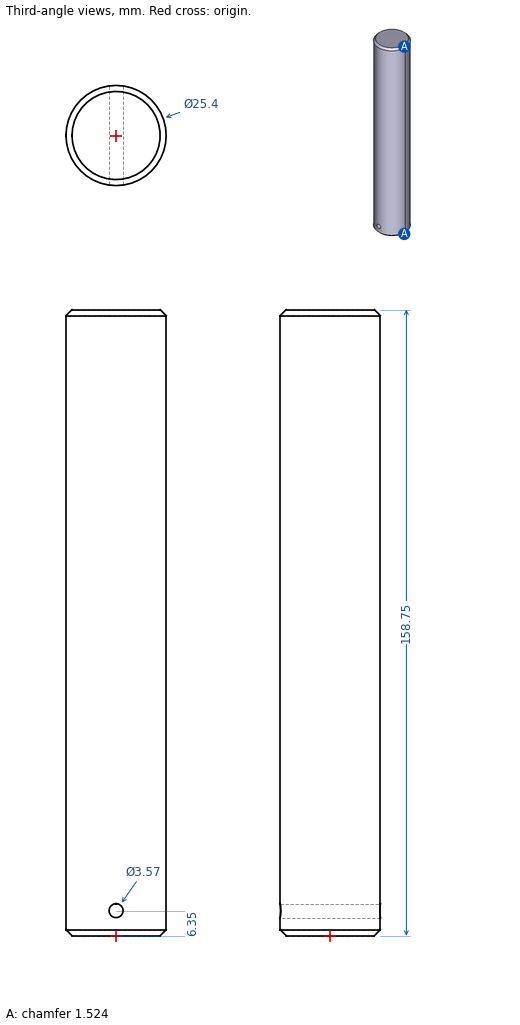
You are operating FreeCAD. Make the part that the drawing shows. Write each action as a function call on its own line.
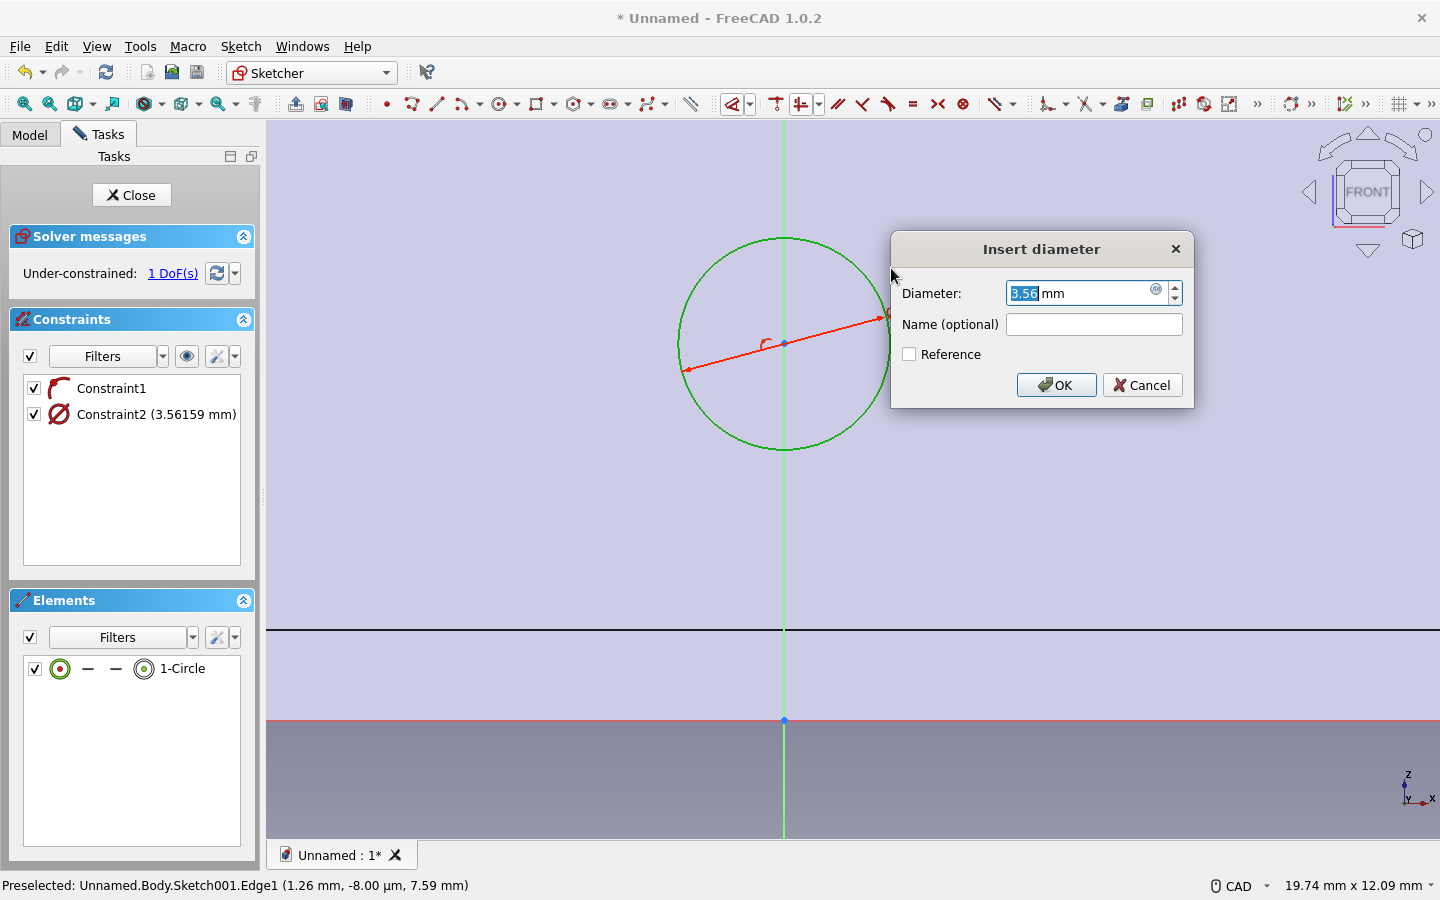
text(3.57)
key(Return)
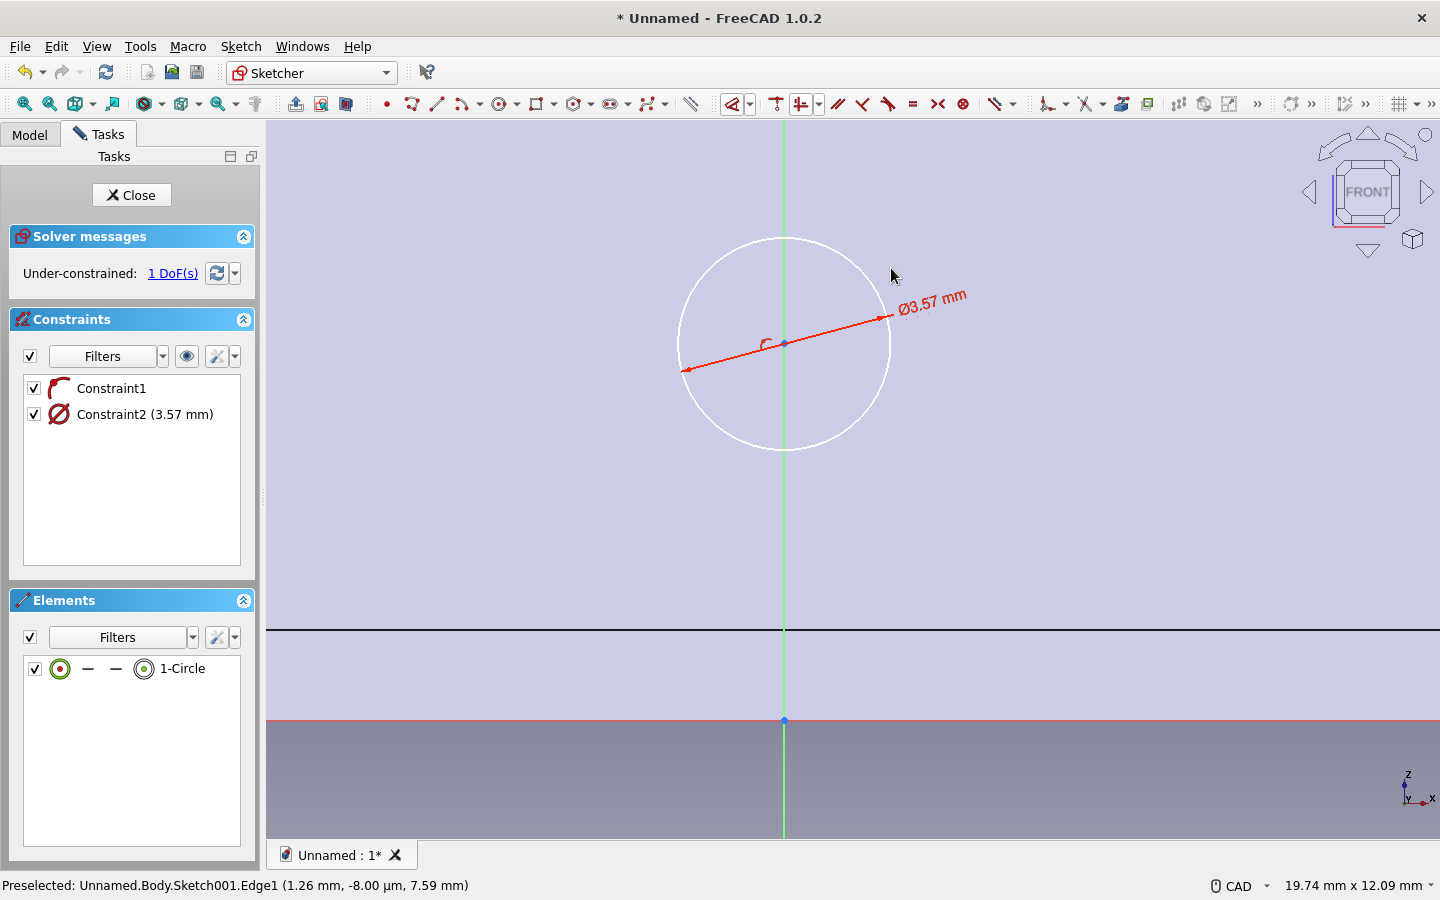
click(784, 344)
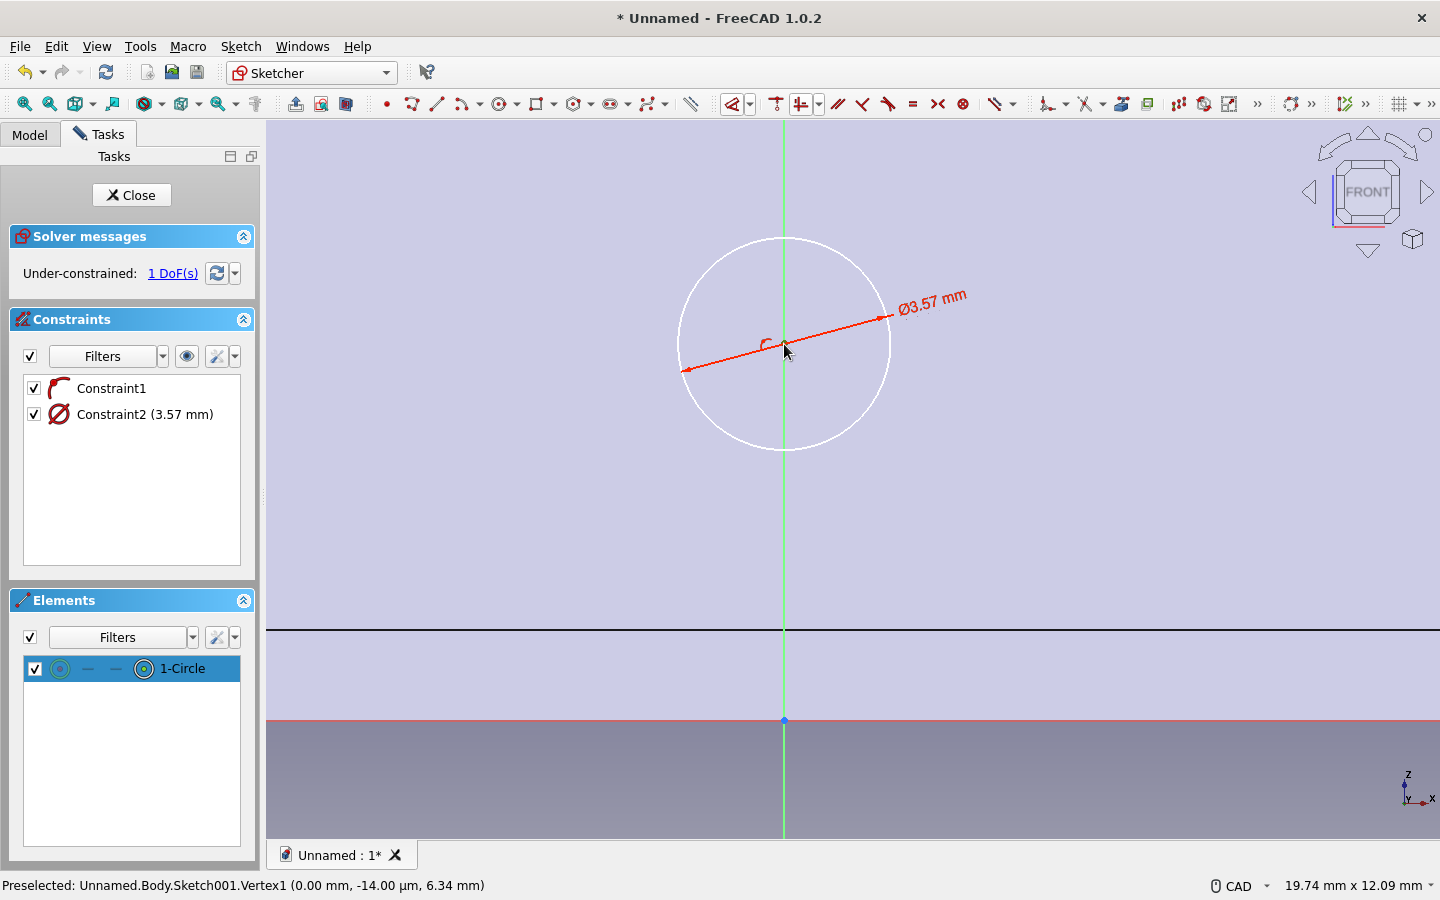
key(i)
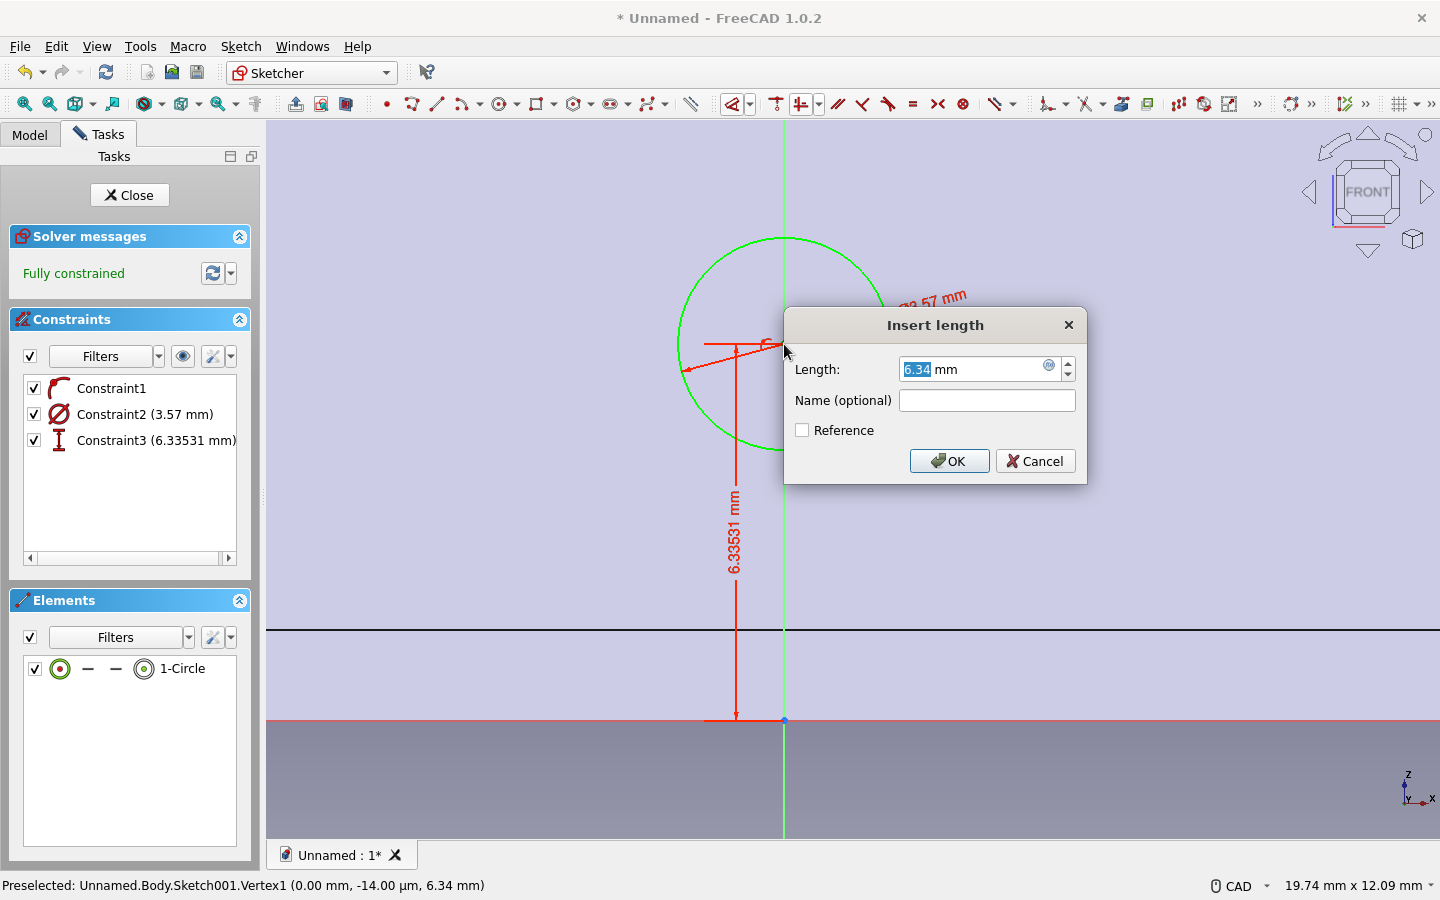
text(6.35)
key(Return)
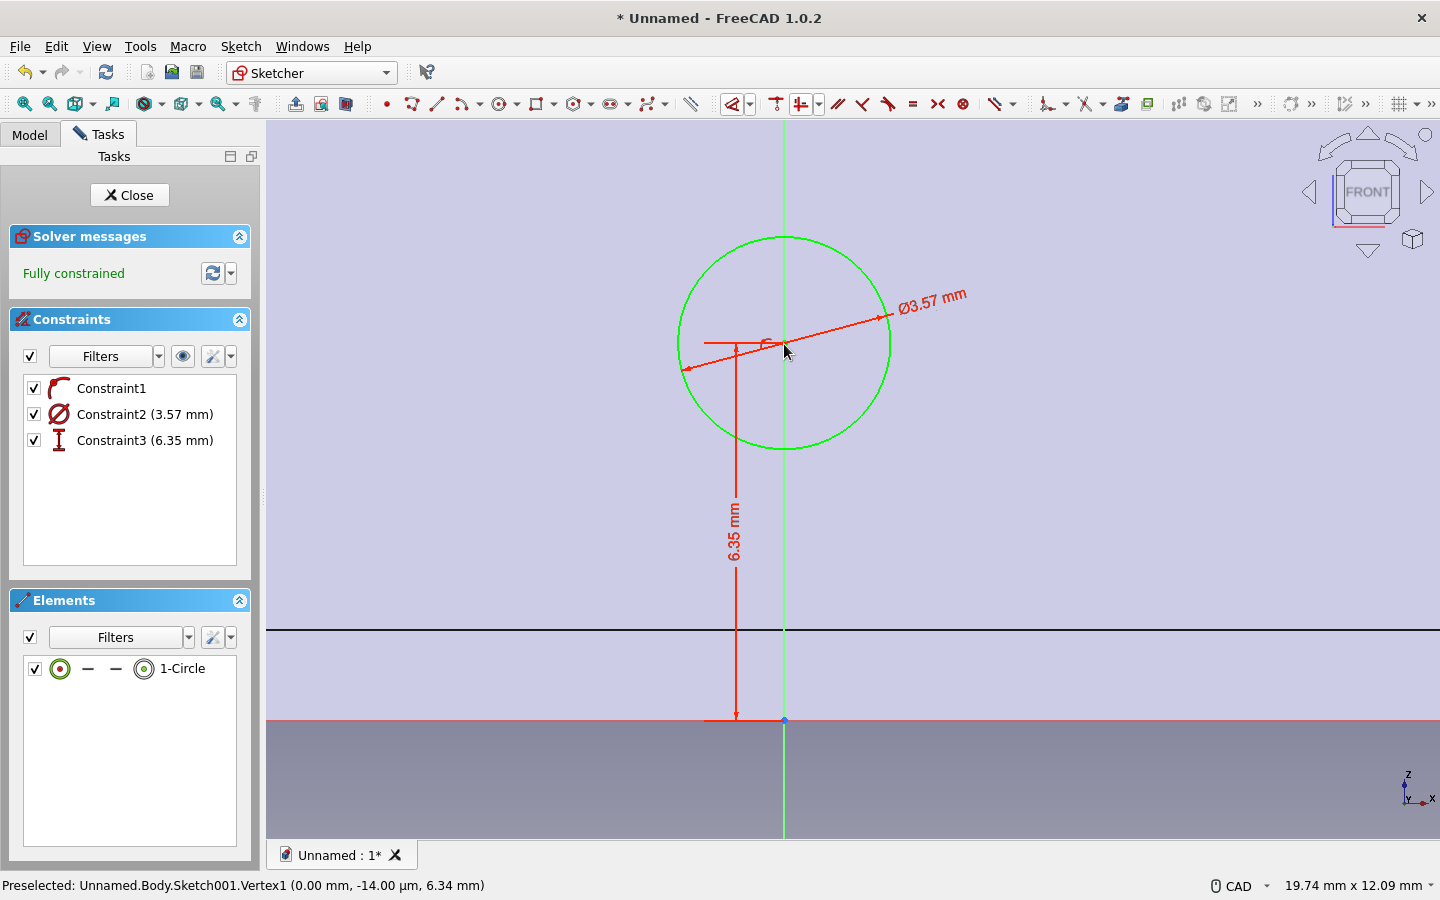
click(130, 195)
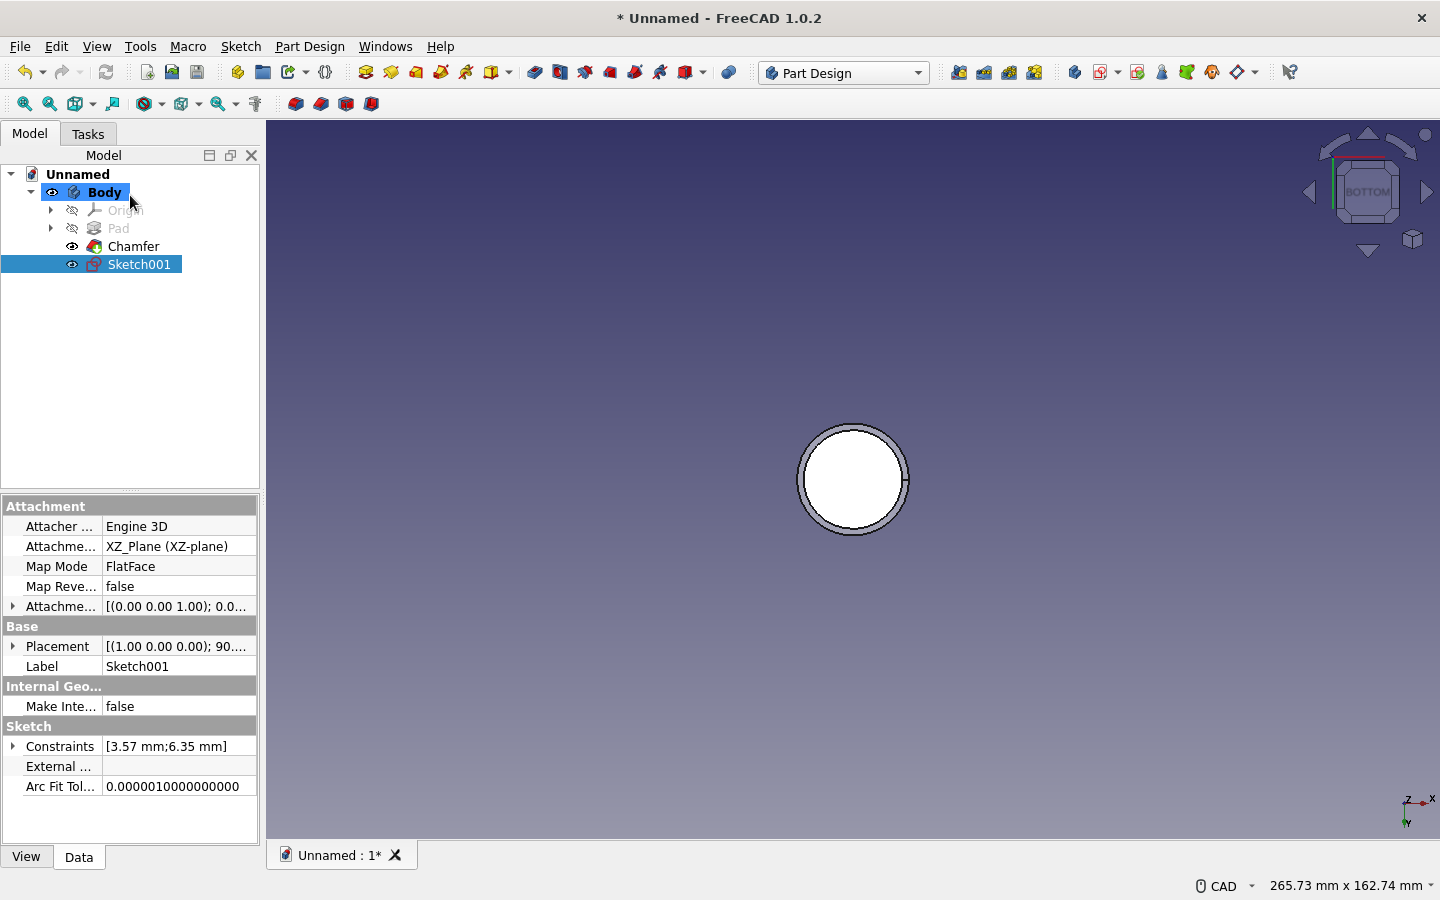
click(535, 72)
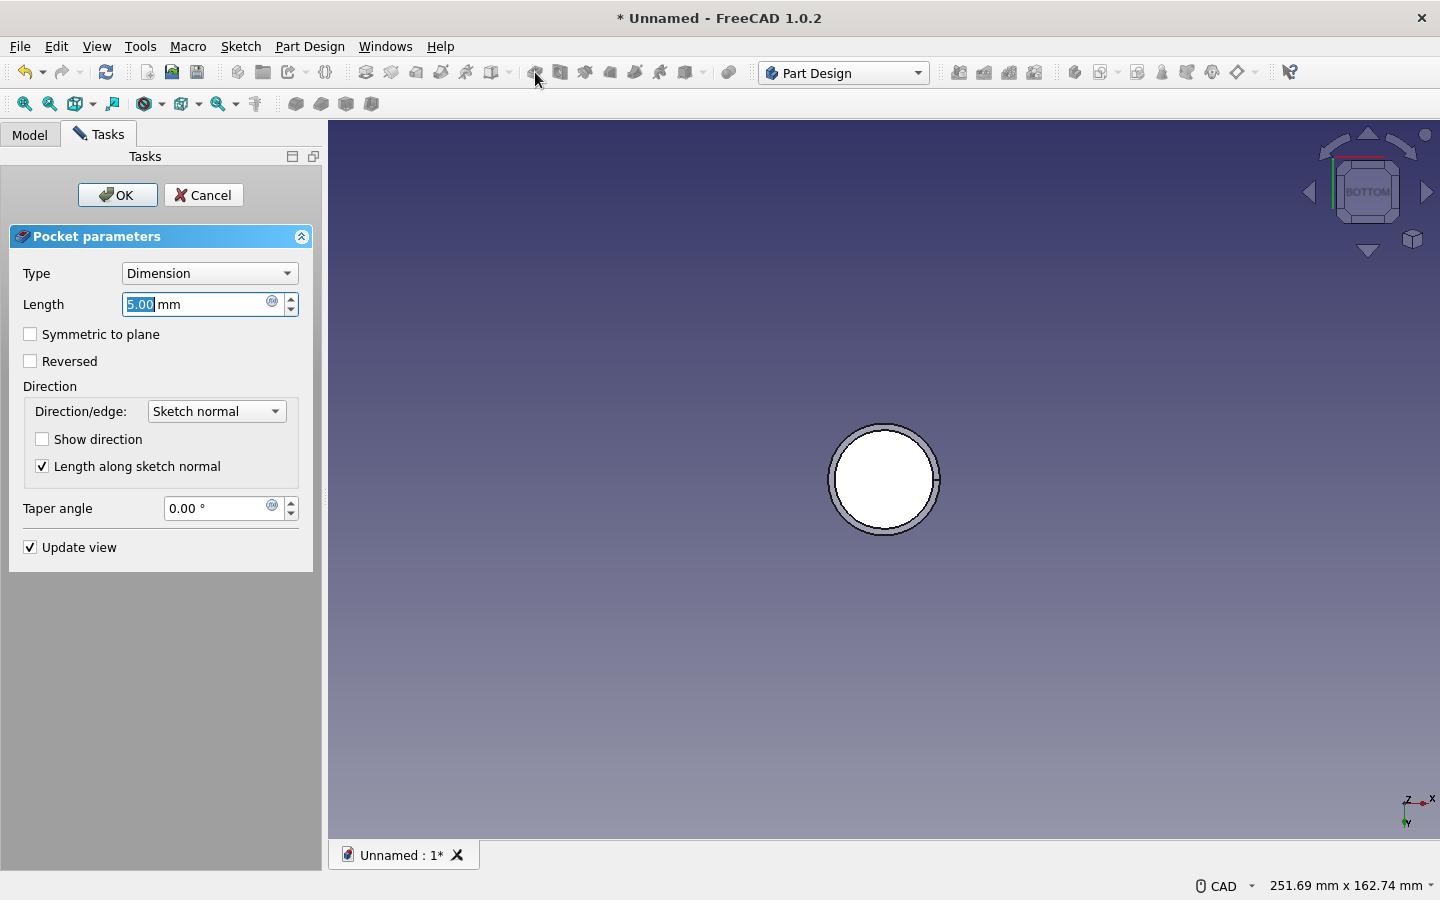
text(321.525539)
key(Tab)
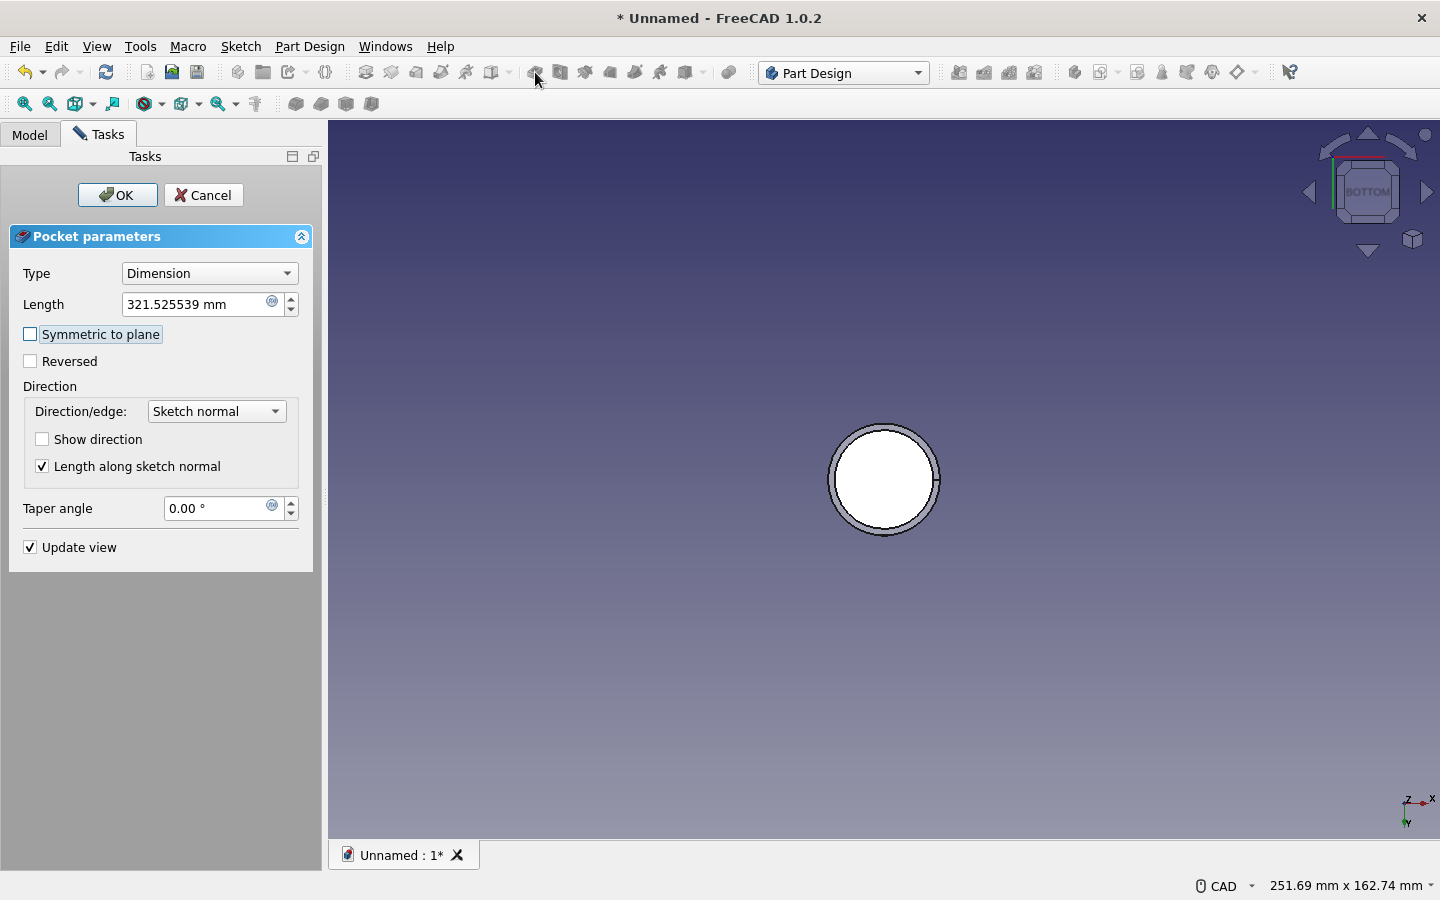
click(31, 334)